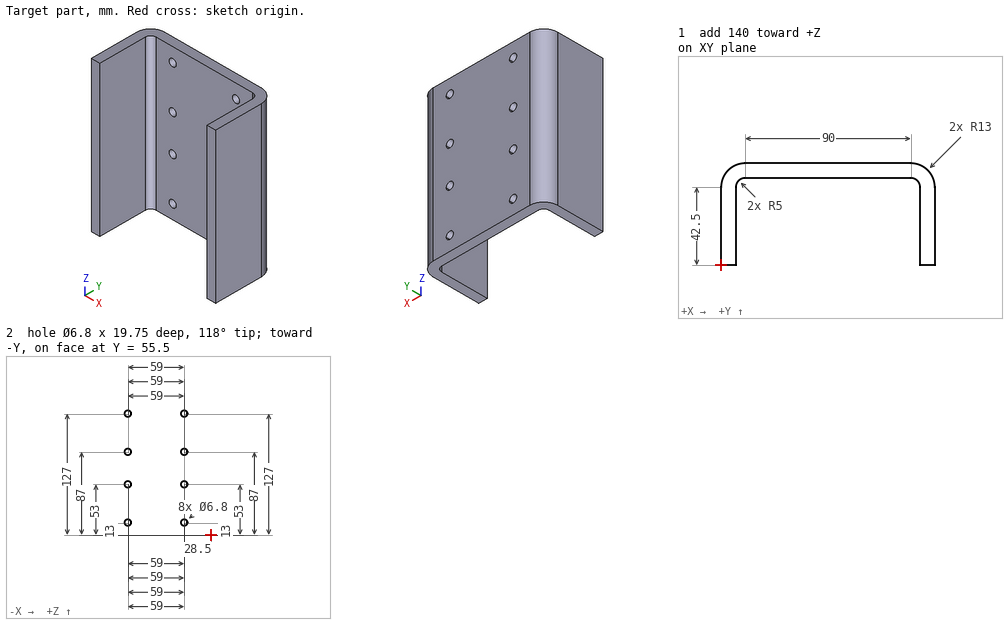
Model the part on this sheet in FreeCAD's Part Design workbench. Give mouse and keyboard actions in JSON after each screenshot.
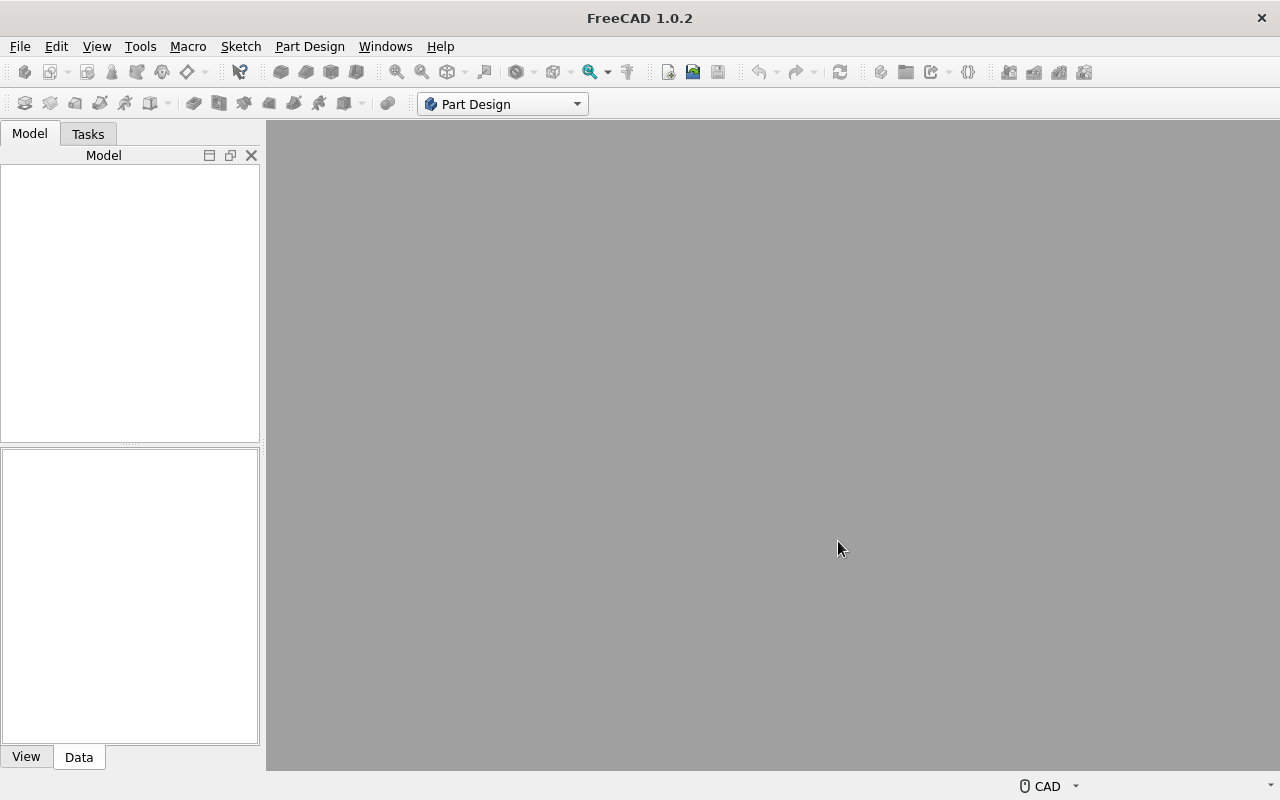
{"action": "left_click", "coordinate": [668, 72]}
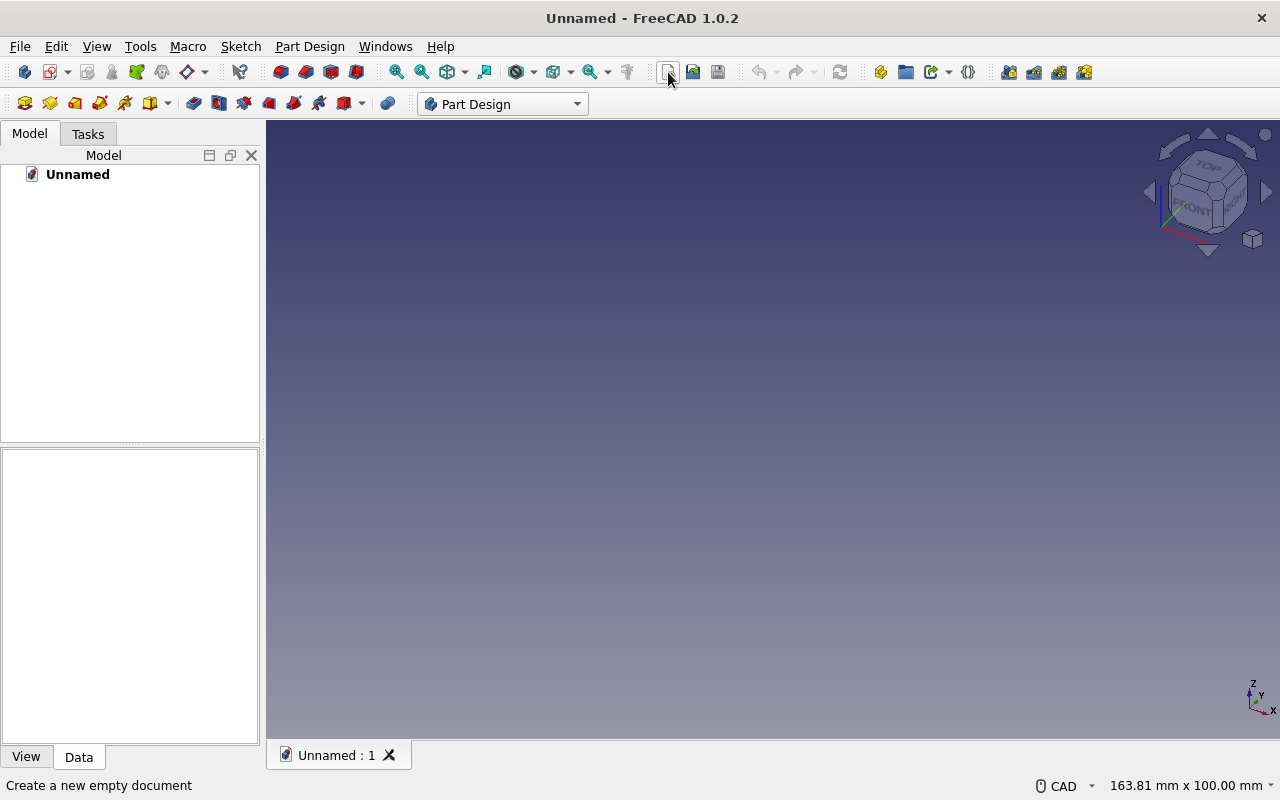
{"action": "left_click", "coordinate": [50, 72]}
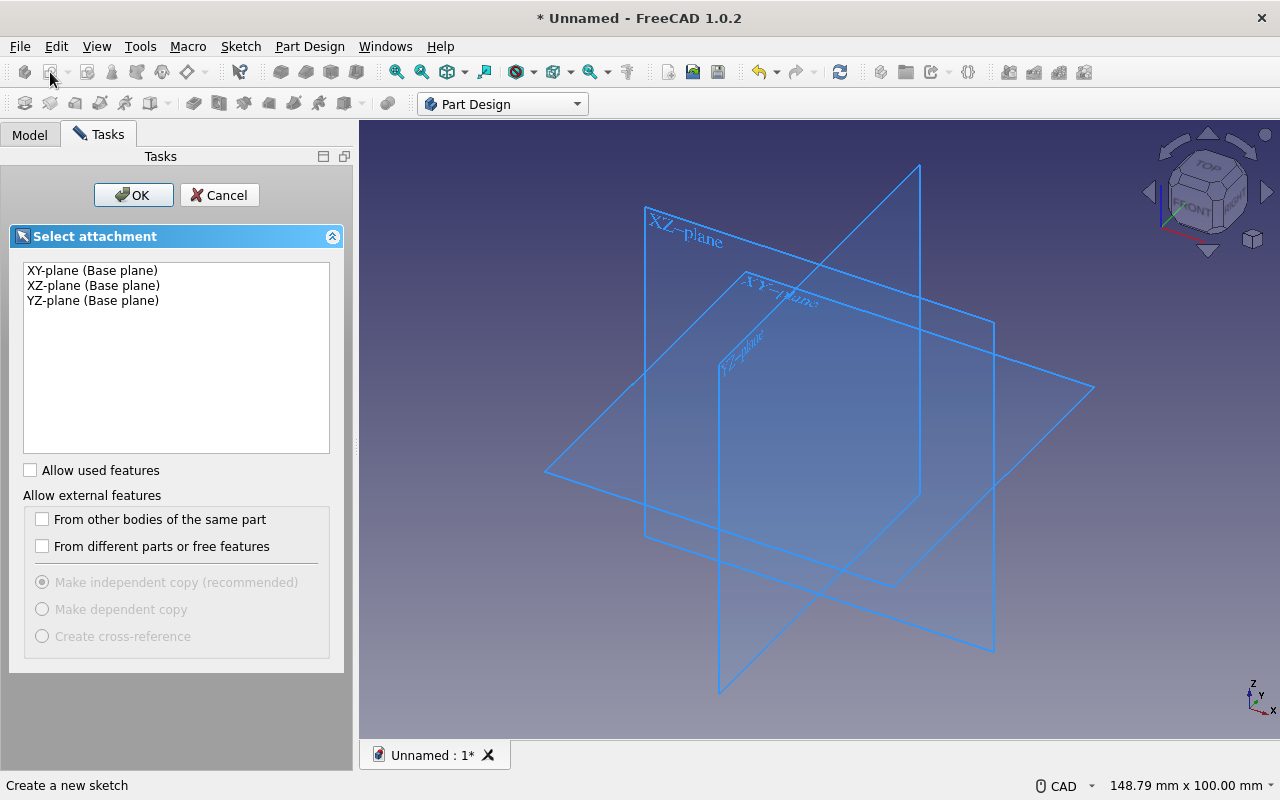
{"action": "left_click", "coordinate": [84, 270]}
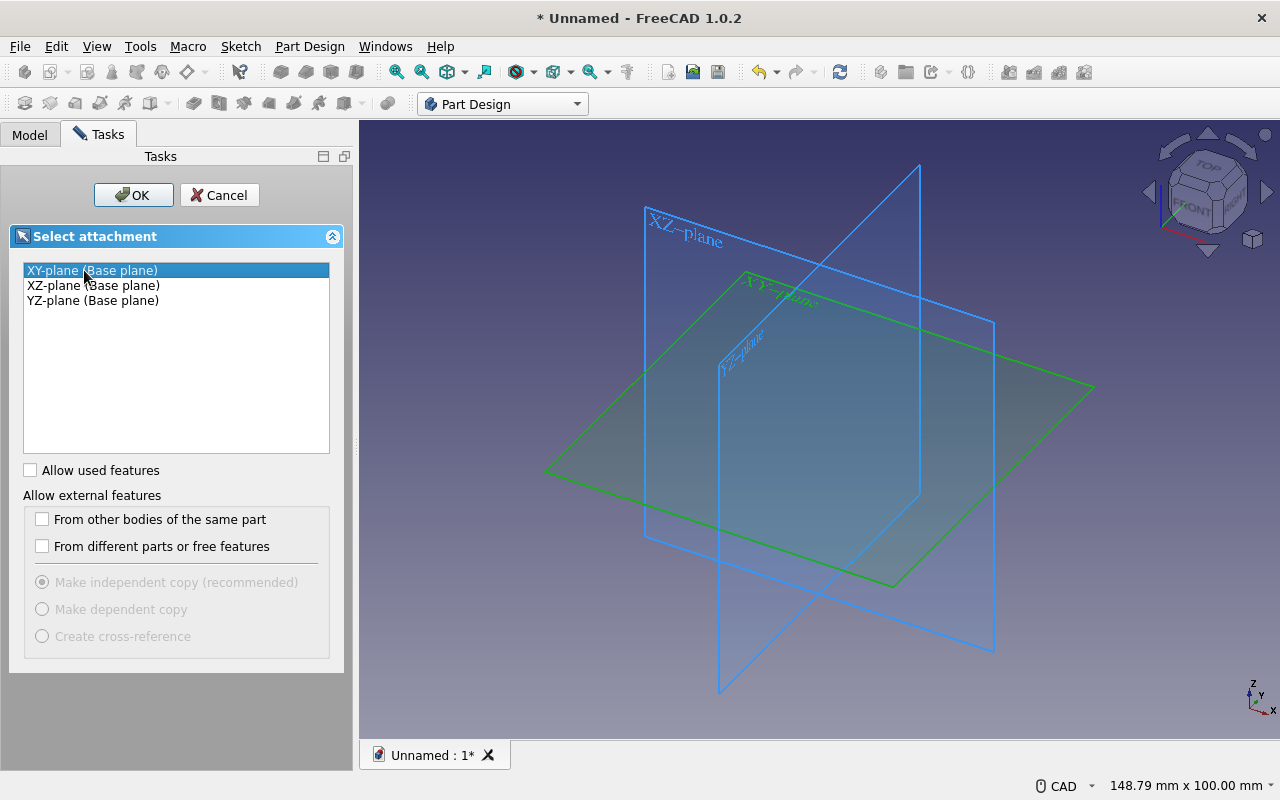
{"action": "left_click", "coordinate": [134, 195]}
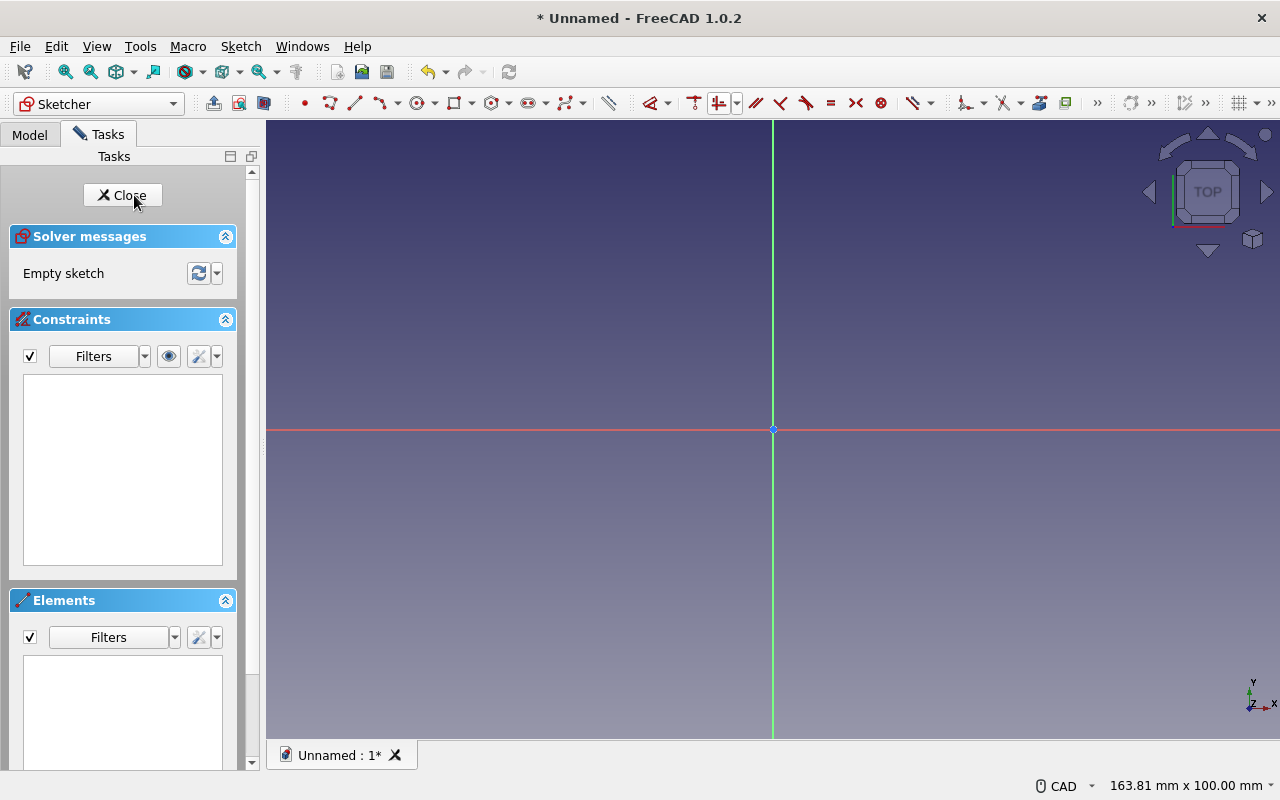
{"action": "scroll", "coordinate": [294, 638], "scroll_direction": "down", "scroll_amount": 3}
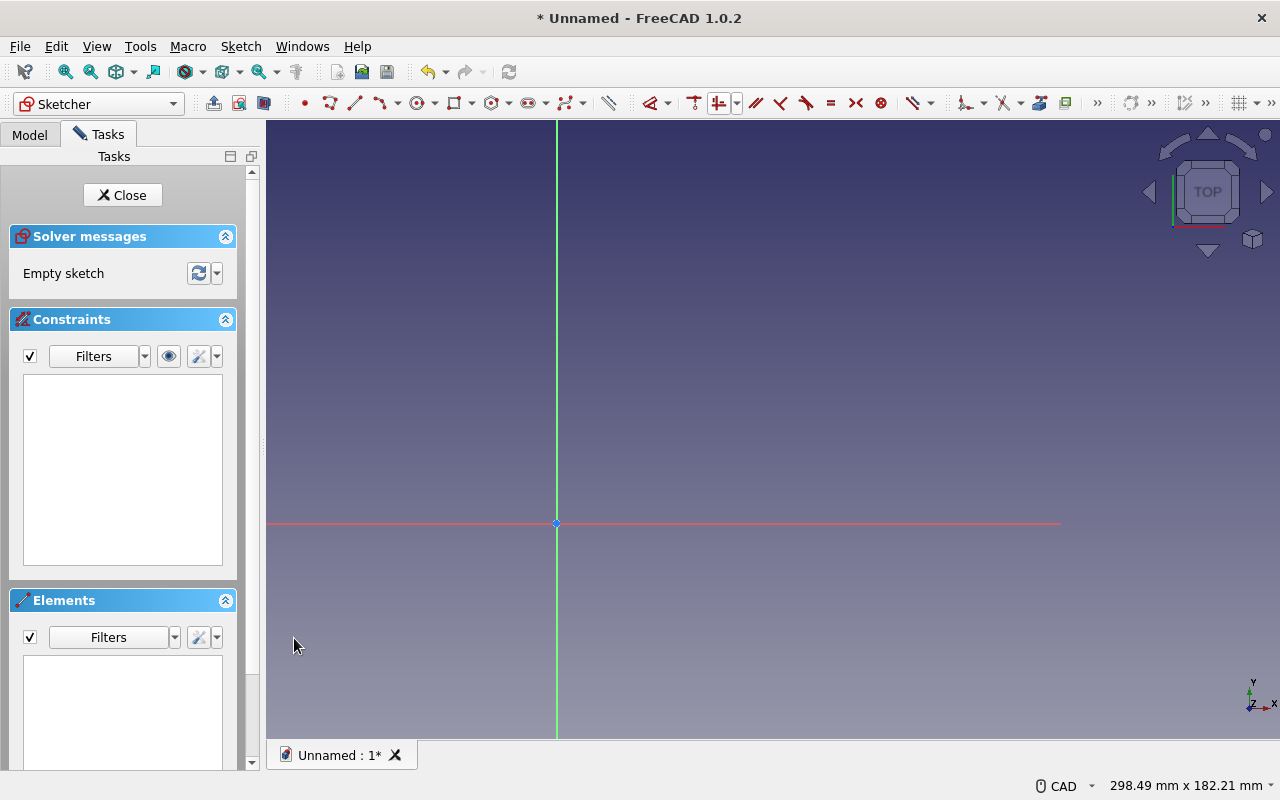
{"action": "scroll", "coordinate": [854, 430], "scroll_direction": "up", "scroll_amount": 2}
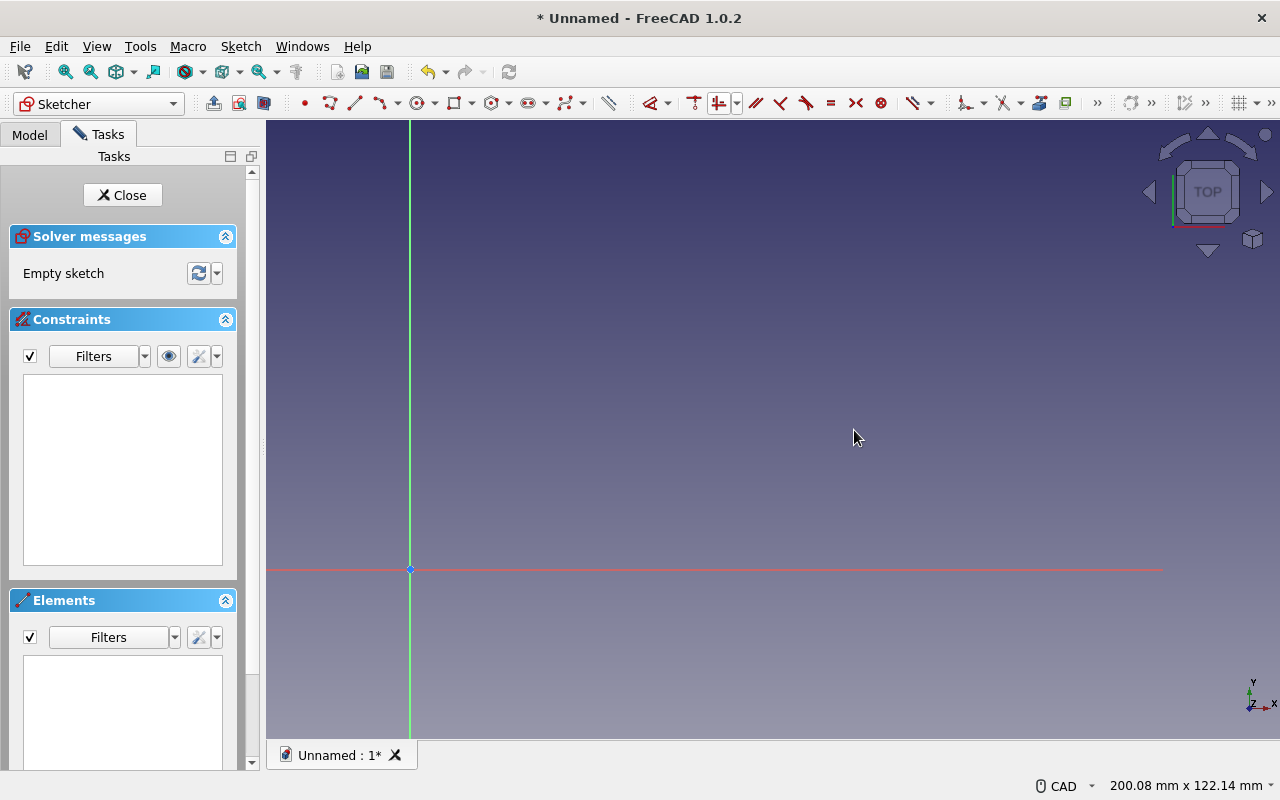
{"action": "key", "text": "g m"}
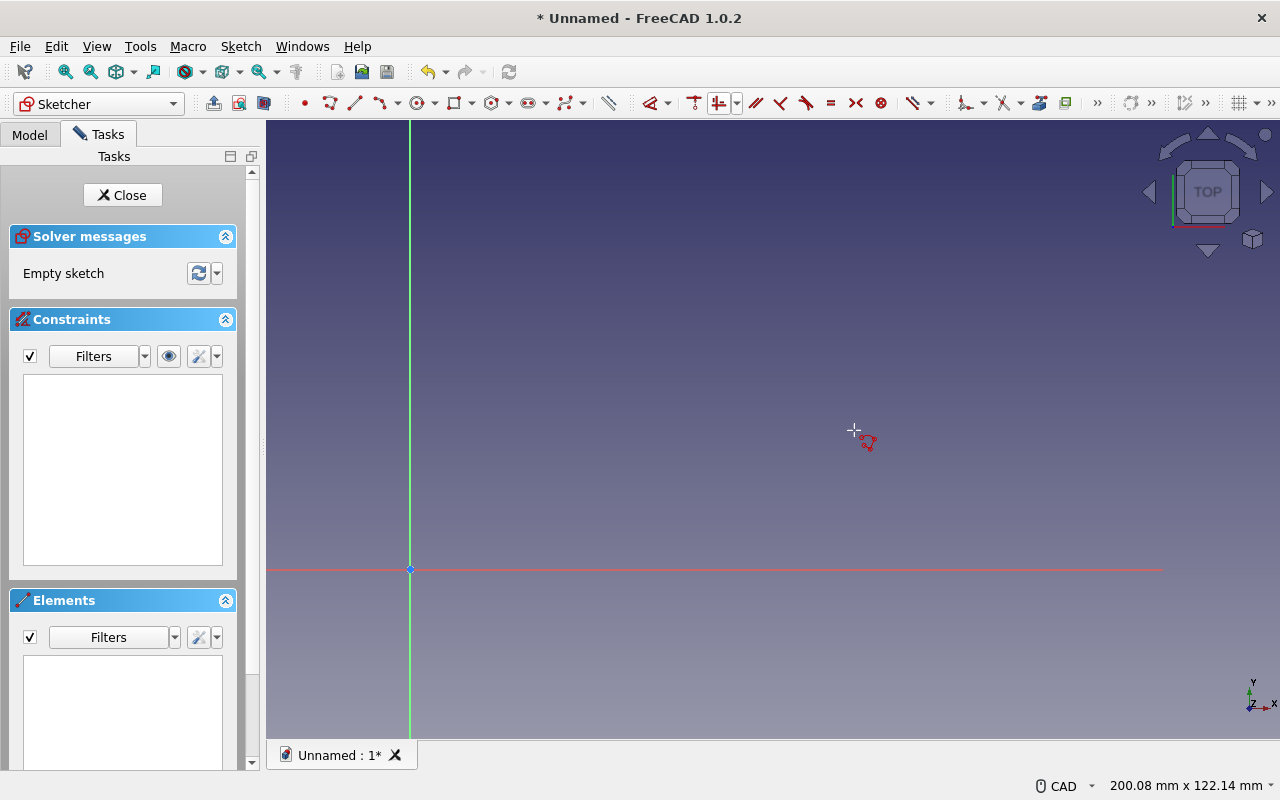
{"action": "left_click", "coordinate": [410, 355]}
{"action": "left_click", "coordinate": [410, 570]}
{"action": "left_click", "coordinate": [451, 561]}
{"action": "left_click", "coordinate": [451, 355]}
{"action": "right_click", "coordinate": [451, 355]}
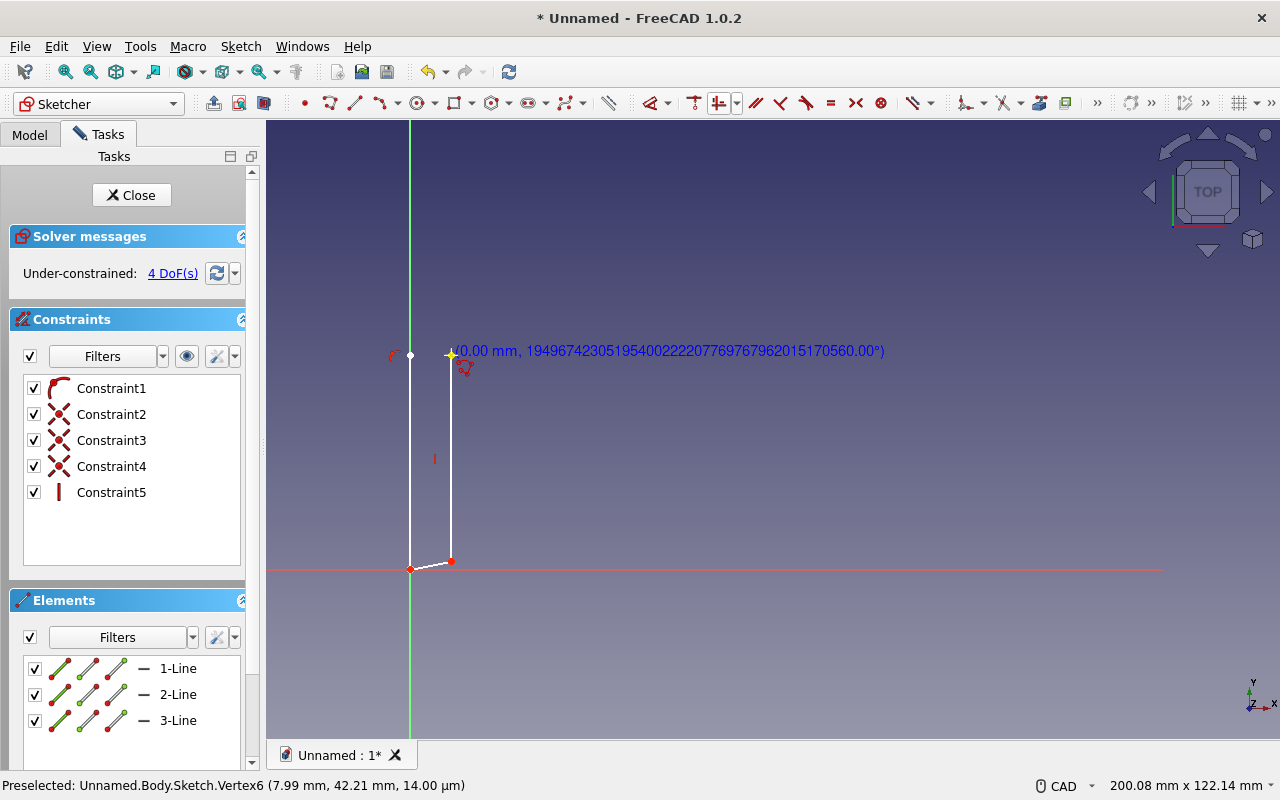
{"action": "key", "text": "g l"}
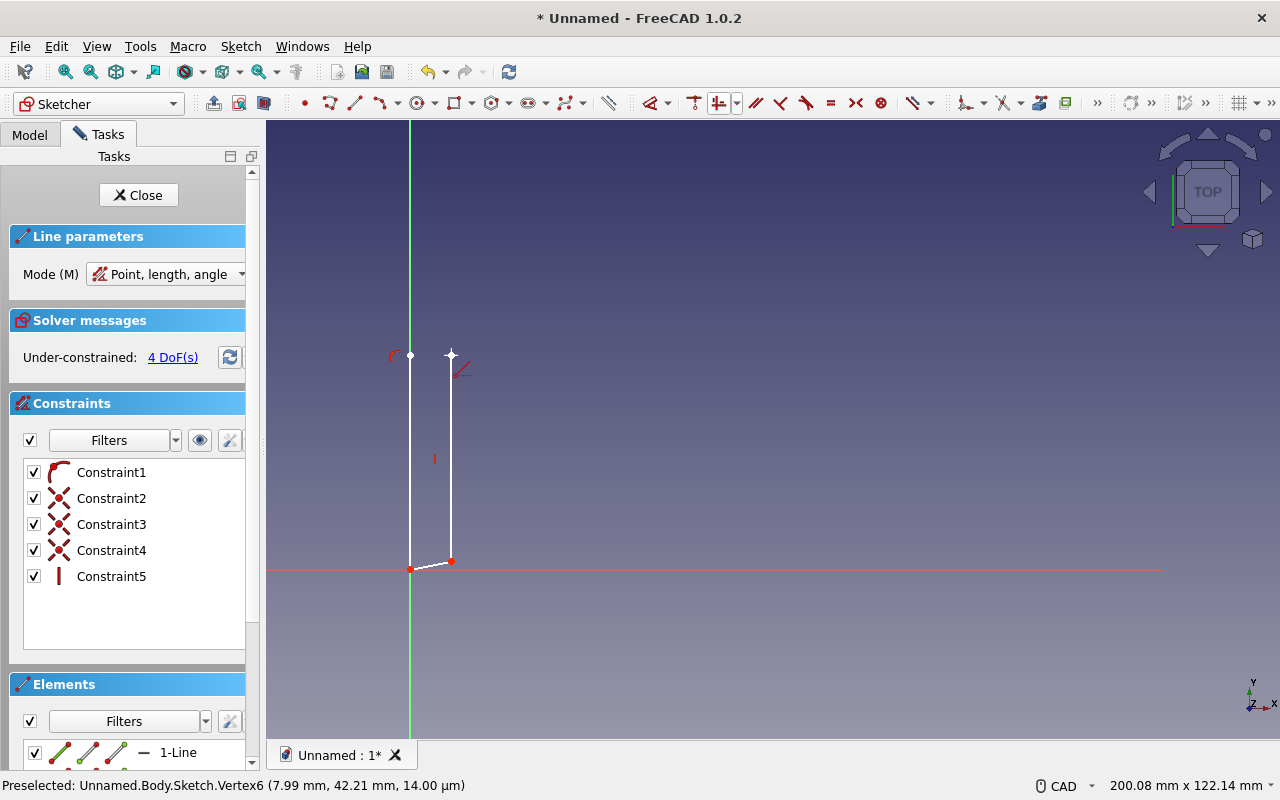
{"action": "left_click", "coordinate": [476, 329]}
{"action": "left_click", "coordinate": [932, 329]}